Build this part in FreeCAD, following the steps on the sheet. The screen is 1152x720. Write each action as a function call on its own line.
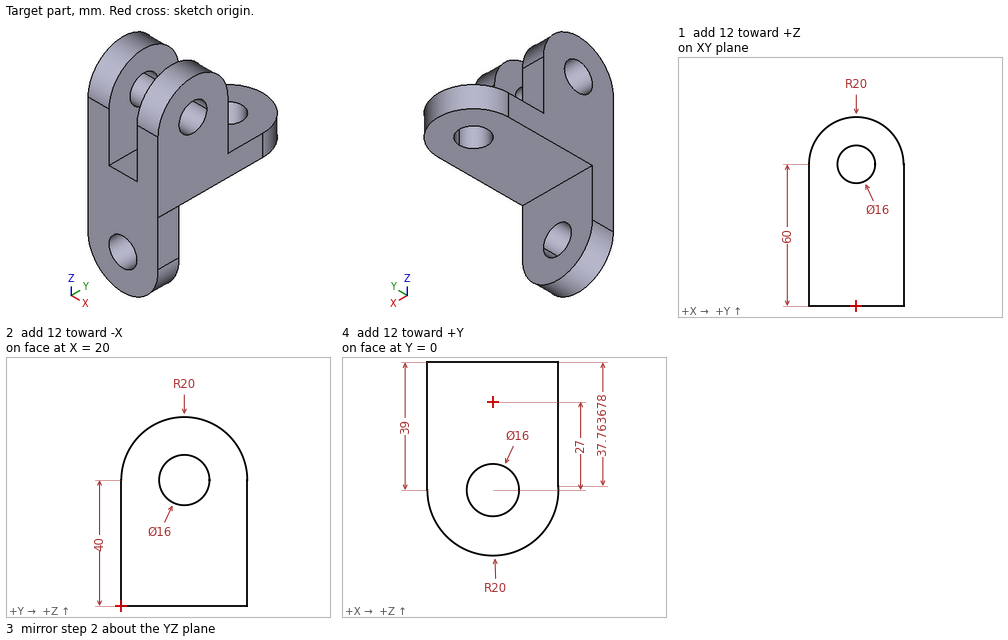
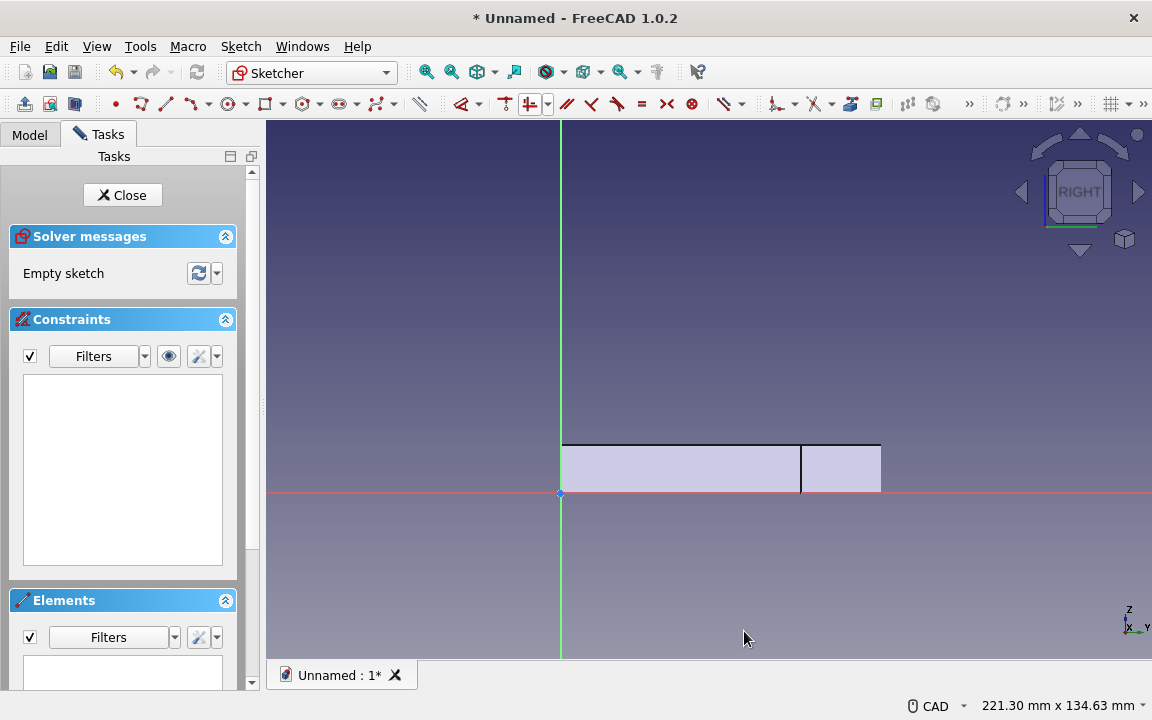
scroll(641, 340, up, 2)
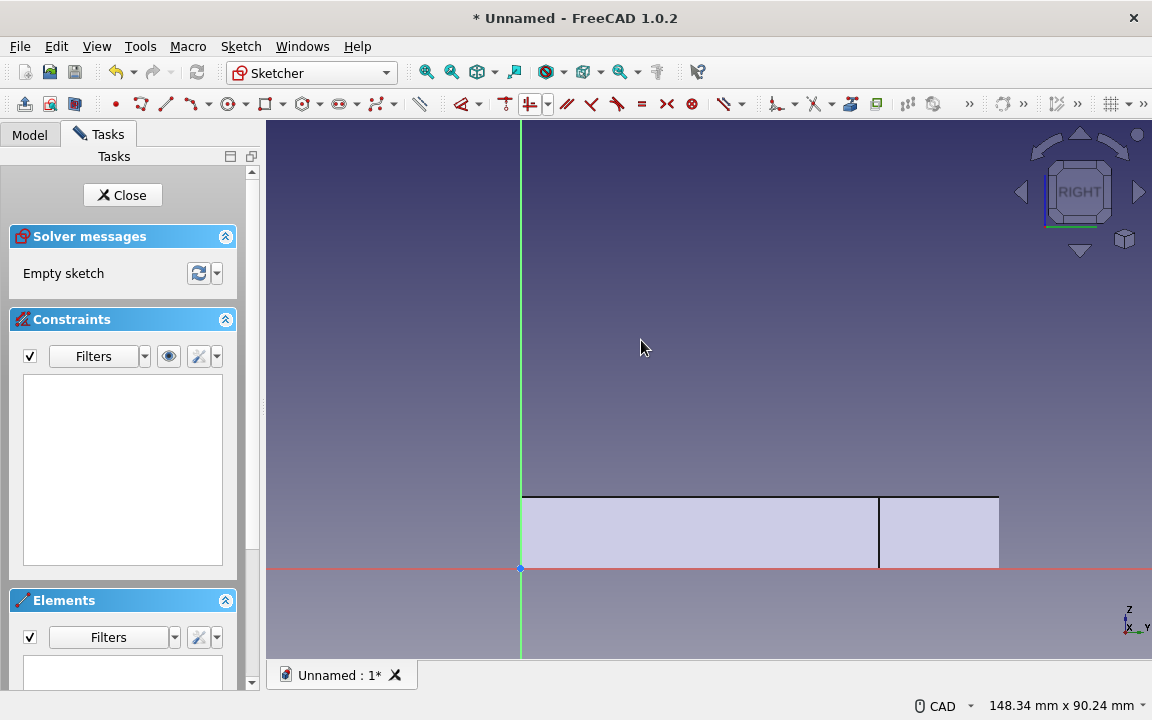
click(141, 104)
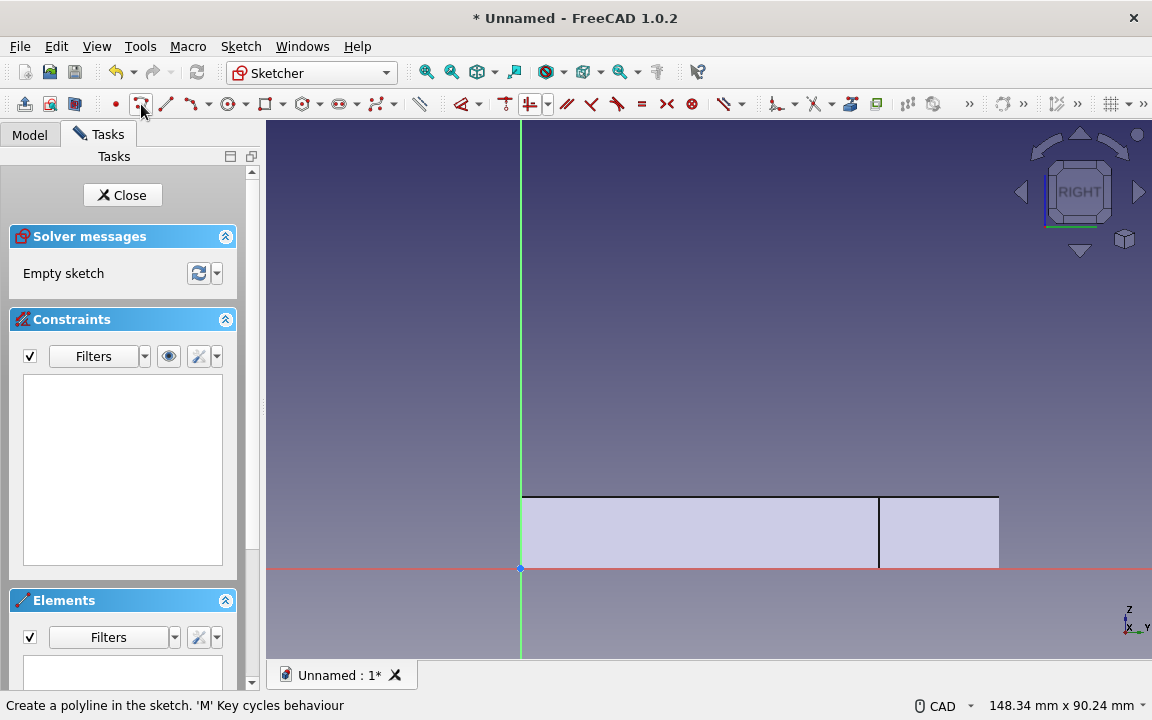
click(521, 330)
click(521, 569)
click(760, 560)
click(760, 330)
right_click(760, 330)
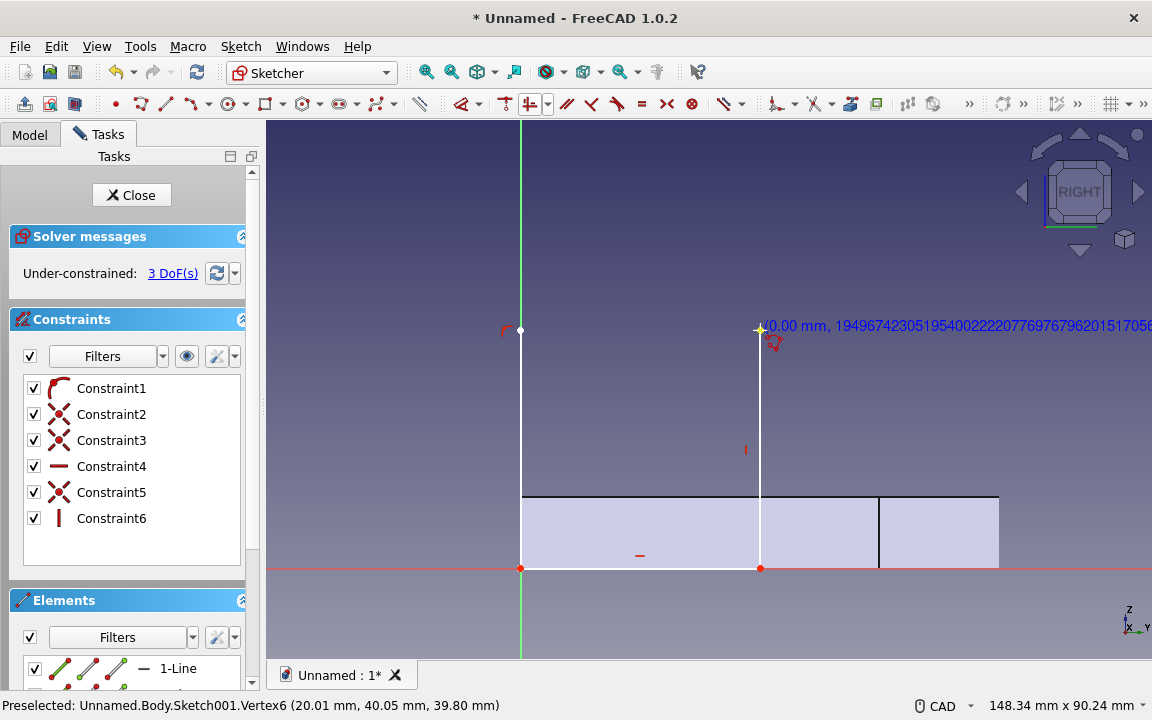
key(g)
key(3)
key(a)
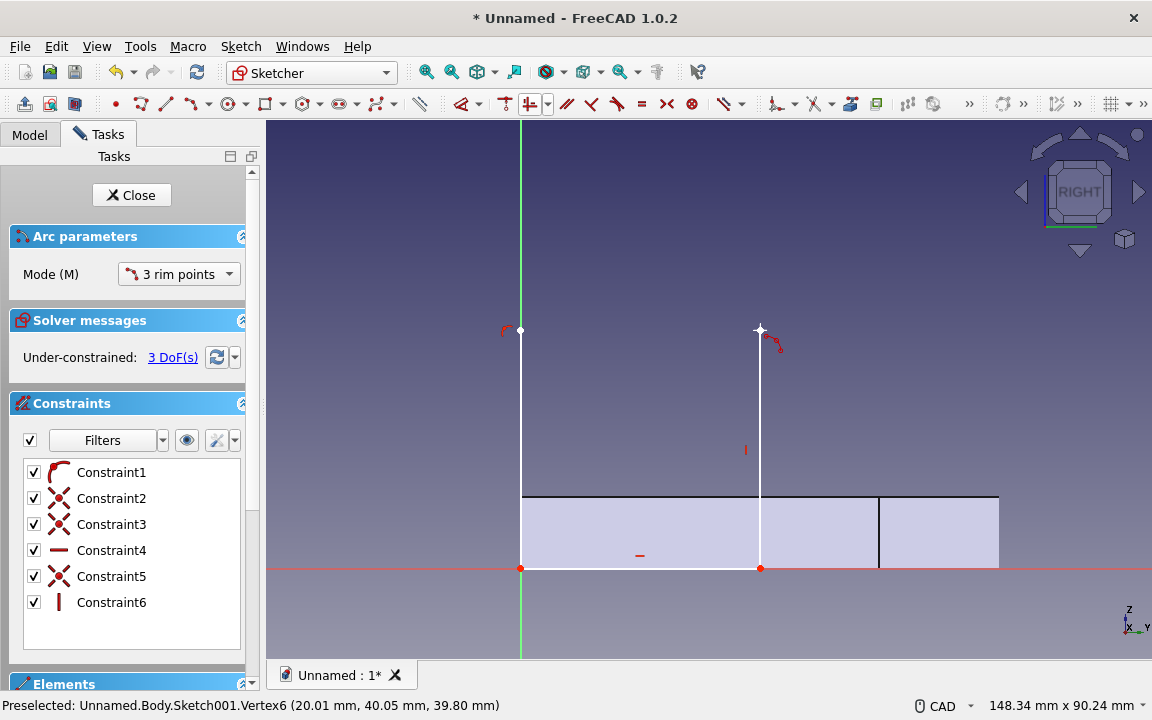
click(760, 331)
click(521, 331)
click(640, 210)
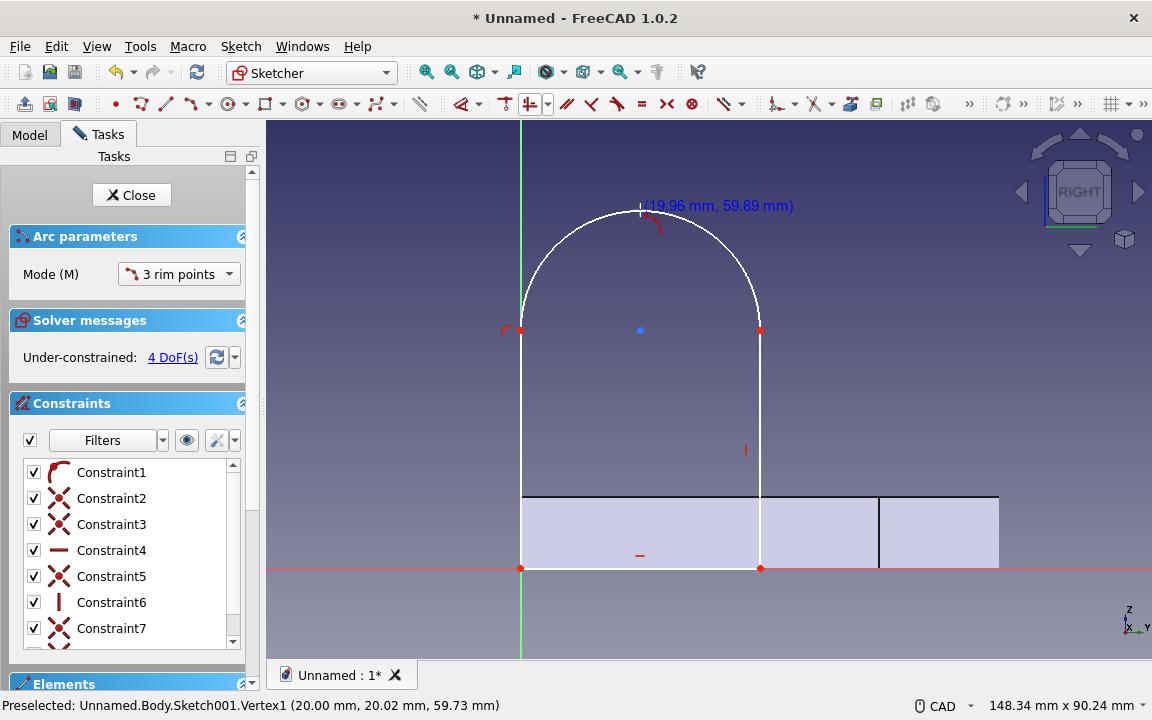
key(g)
key(c)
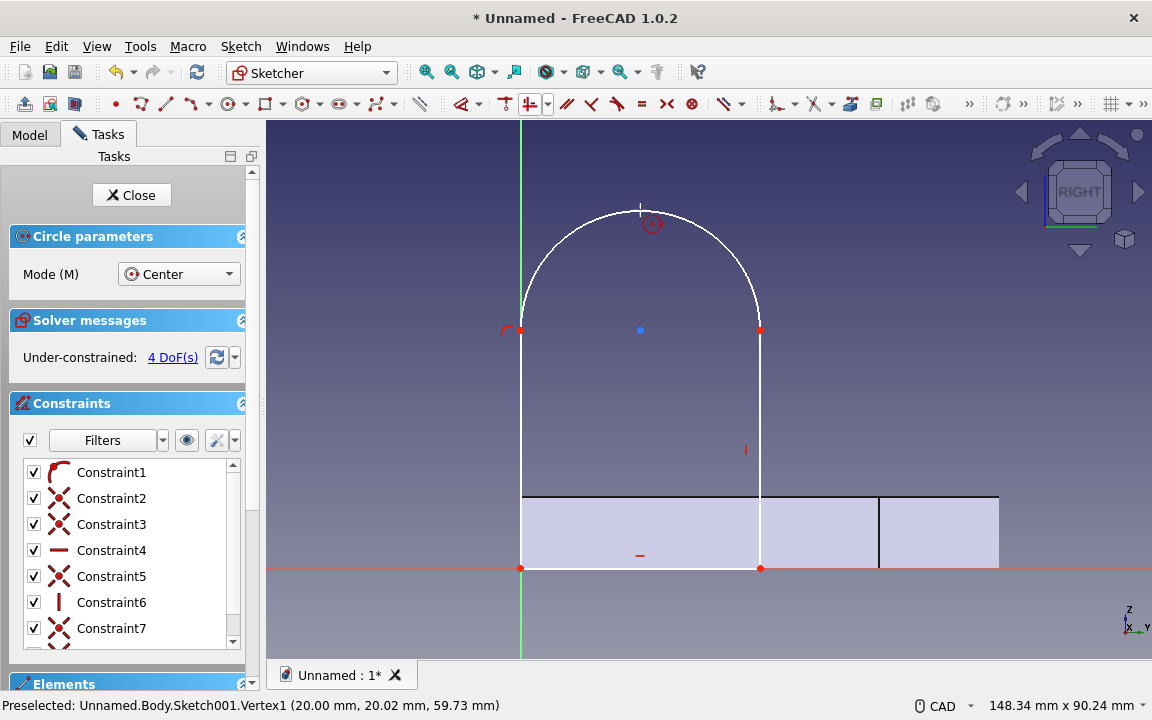
click(640, 330)
move(674, 296)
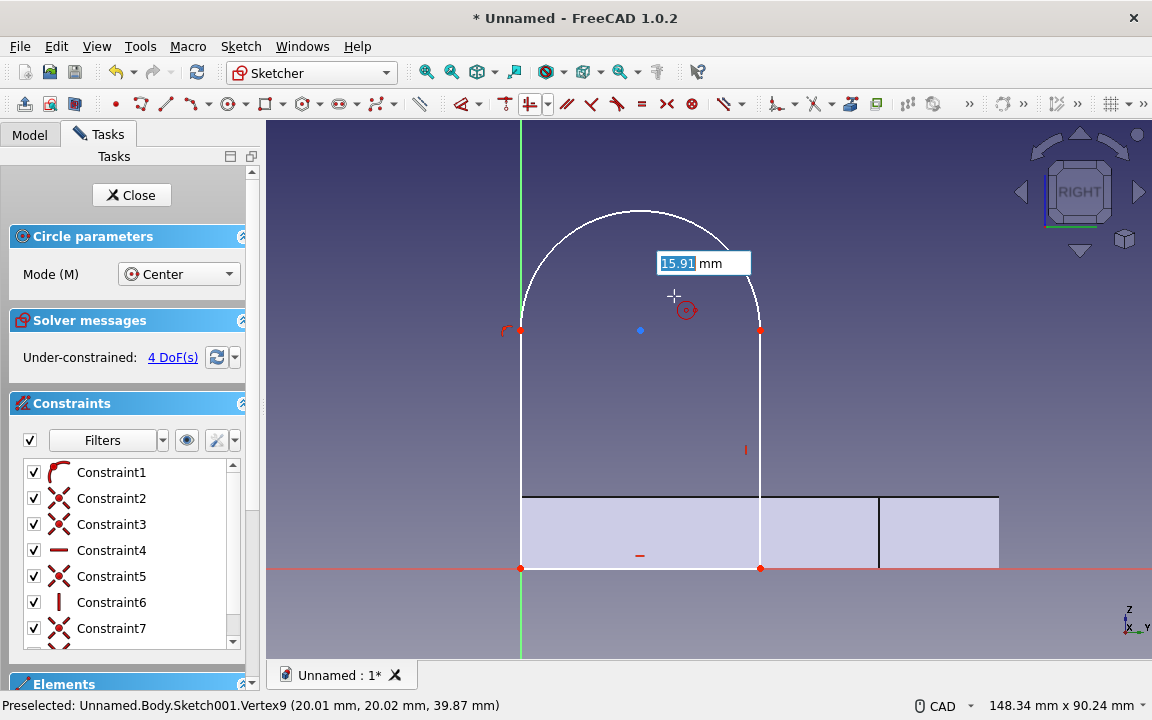
text(16)
key(Return)
key(Escape)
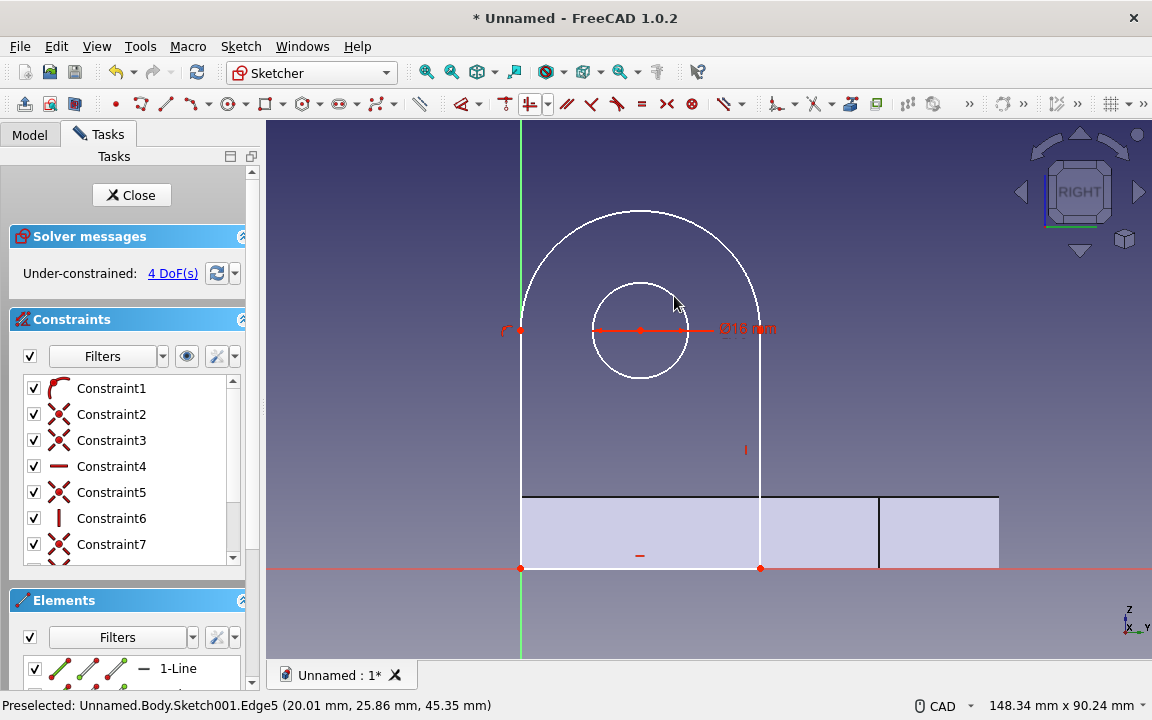
click(521, 402)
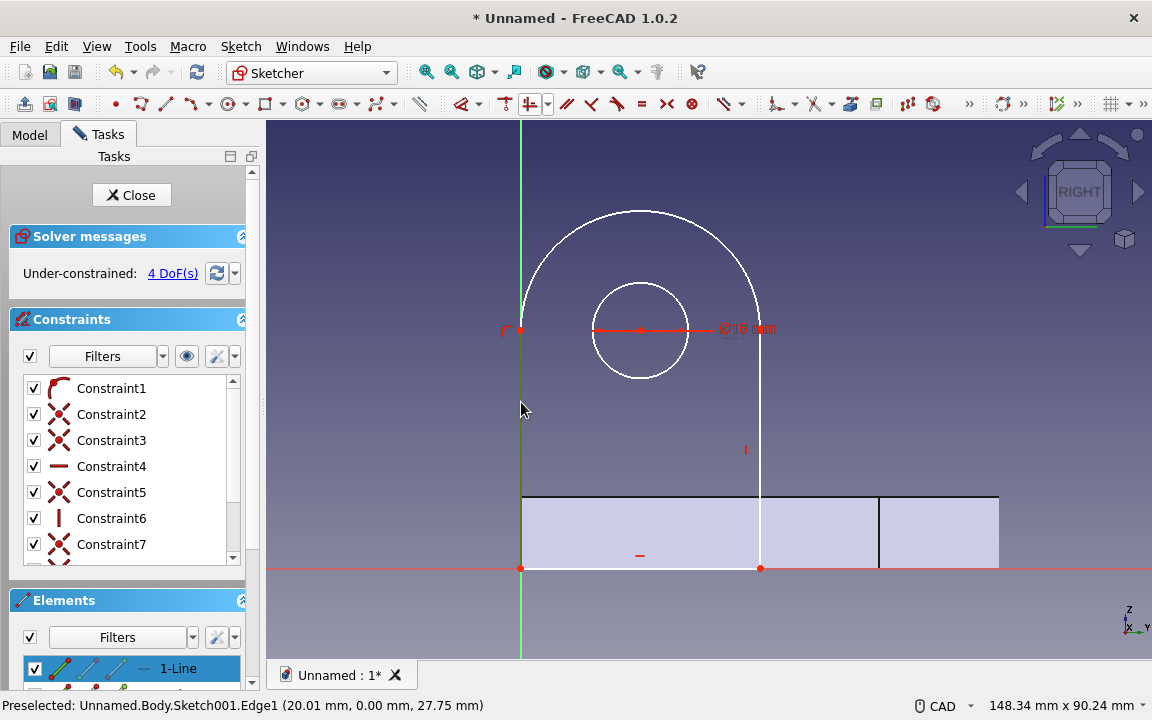
click(711, 234)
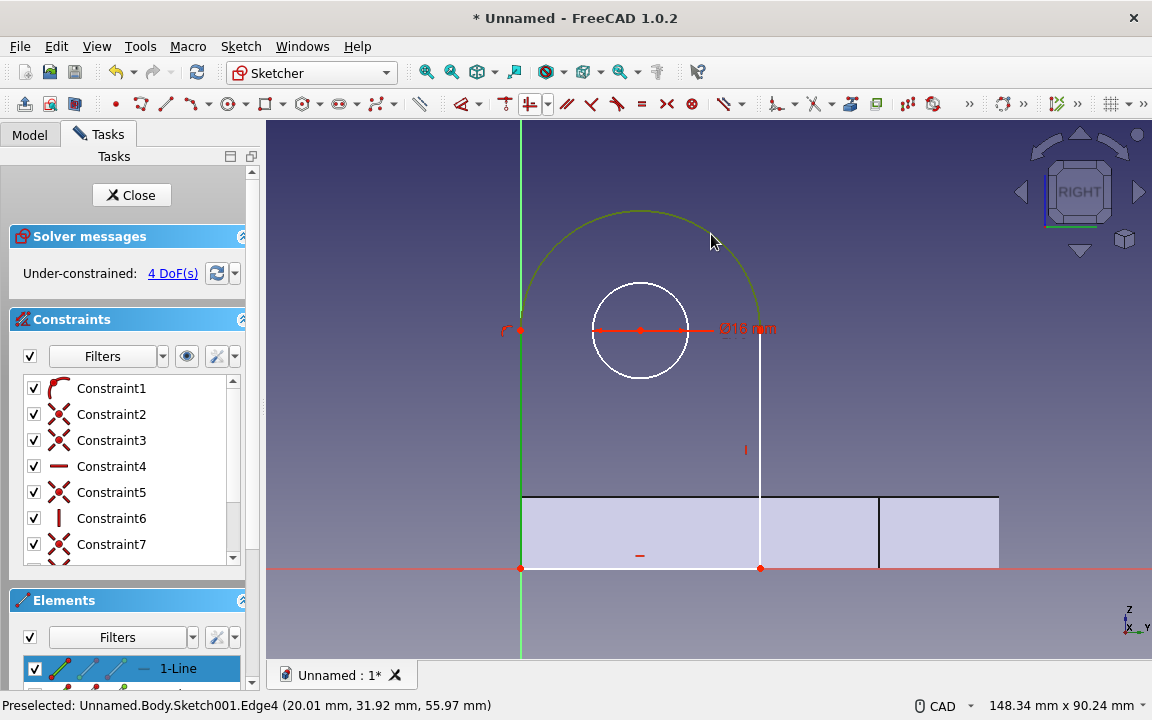
key(t)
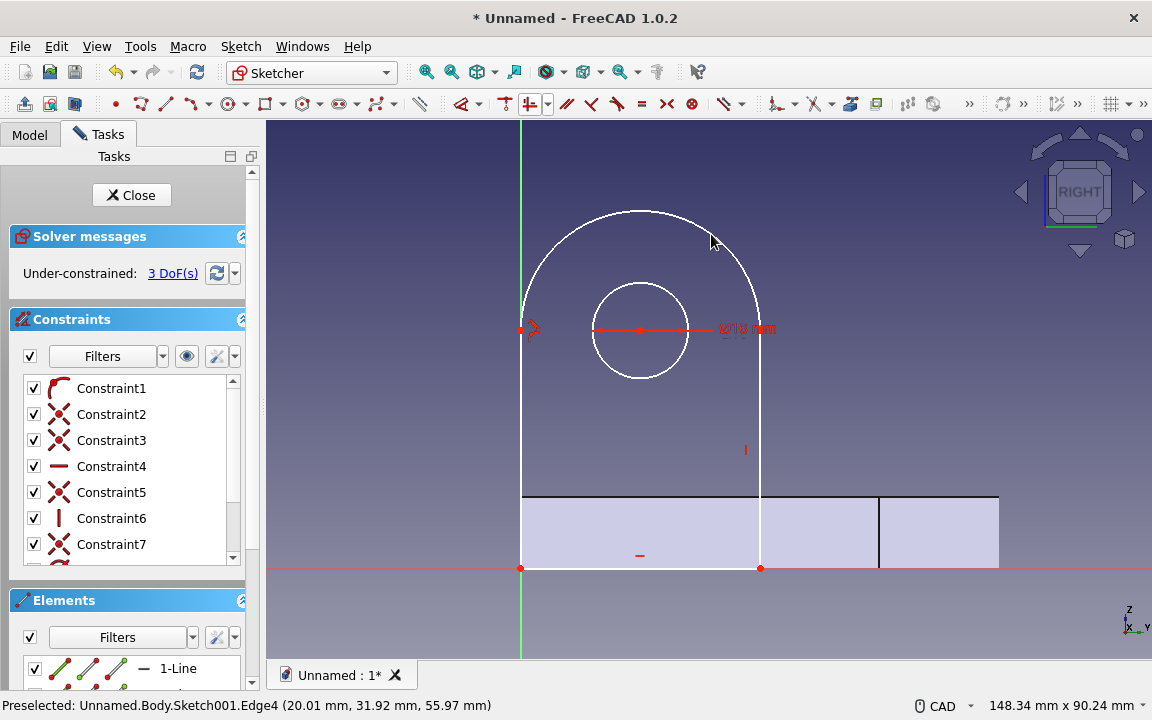
click(760, 497)